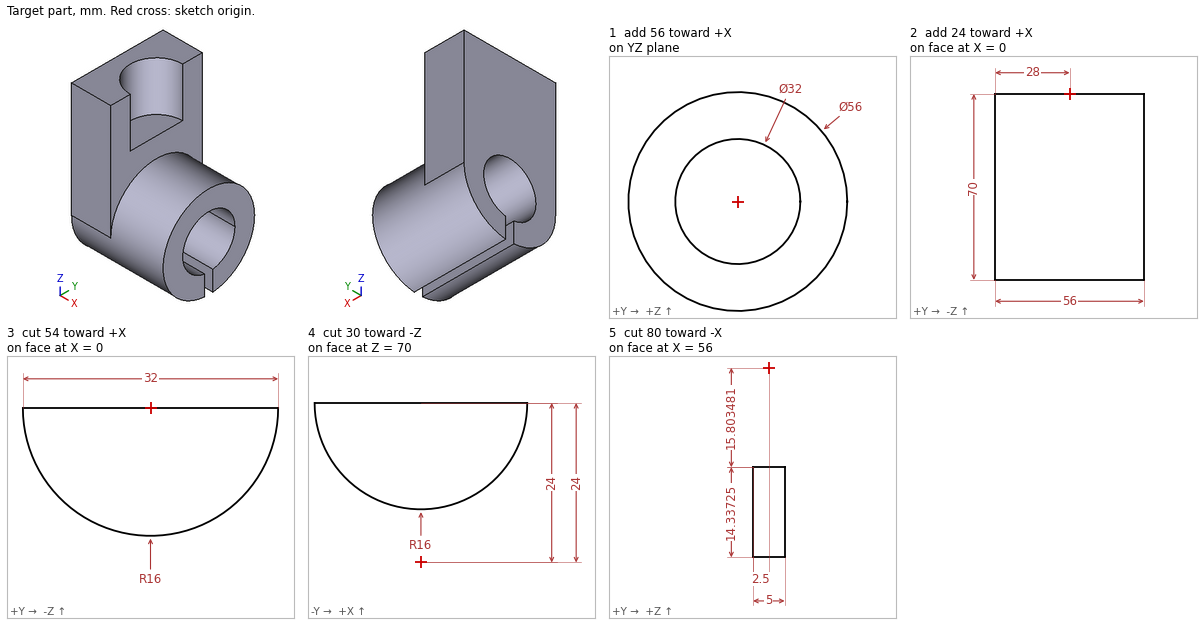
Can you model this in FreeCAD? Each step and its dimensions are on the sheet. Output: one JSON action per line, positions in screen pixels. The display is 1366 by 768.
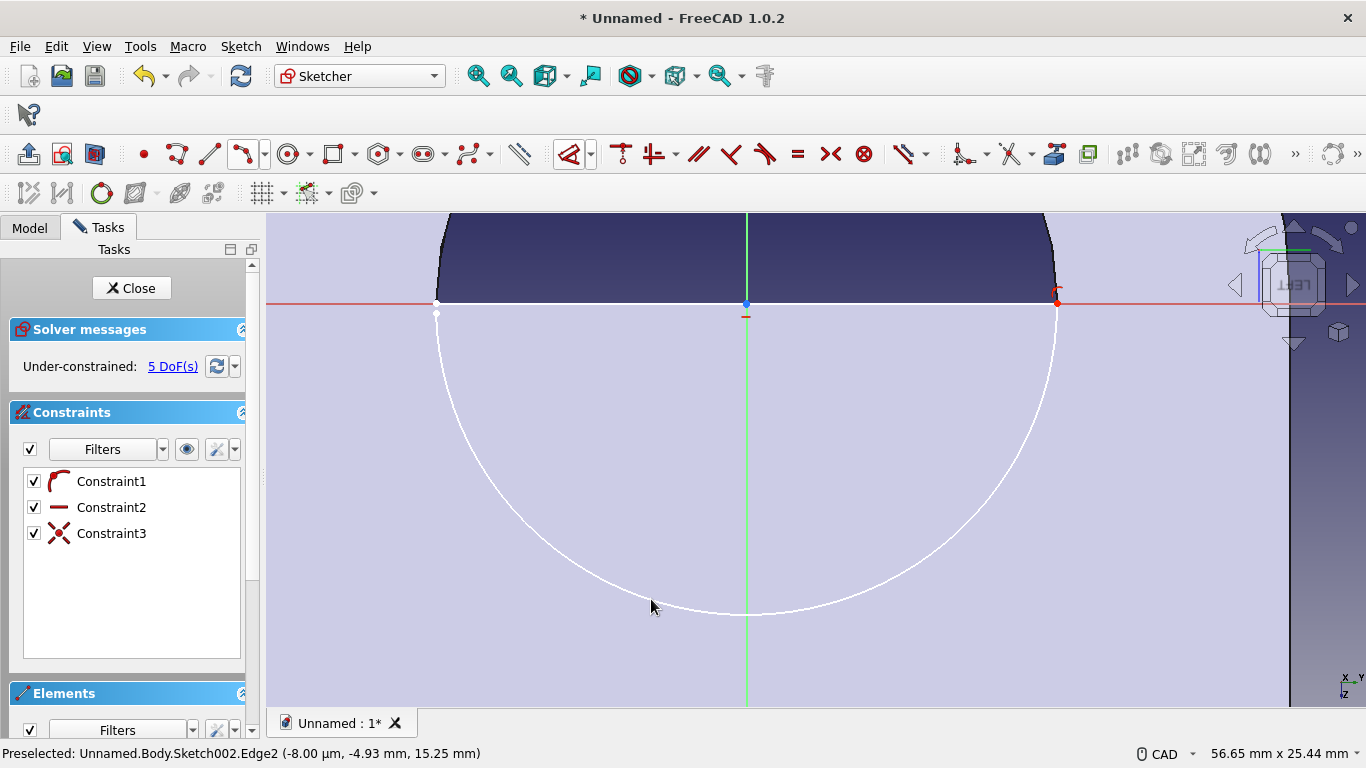
{"action": "left_click_drag", "start_coordinate": [736, 294], "coordinate": [757, 314]}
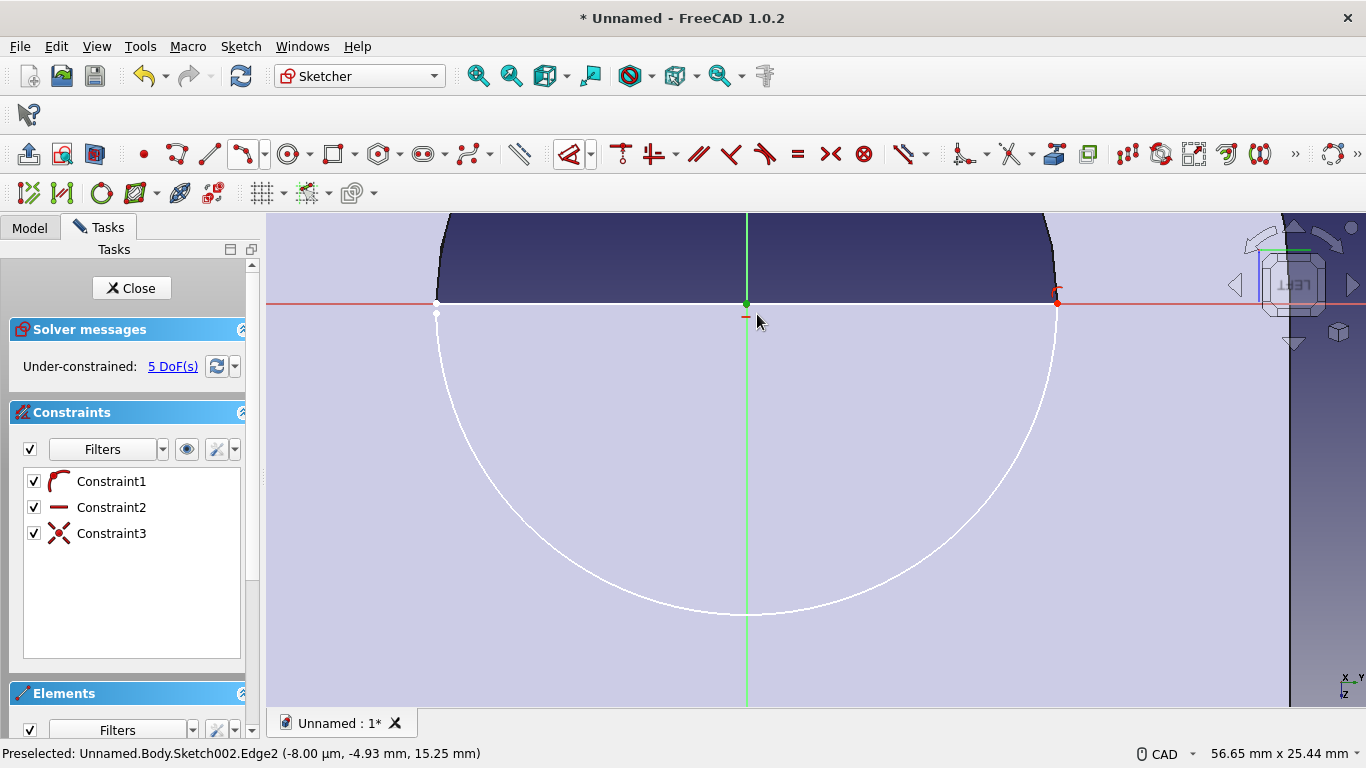
{"action": "left_click", "coordinate": [621, 154]}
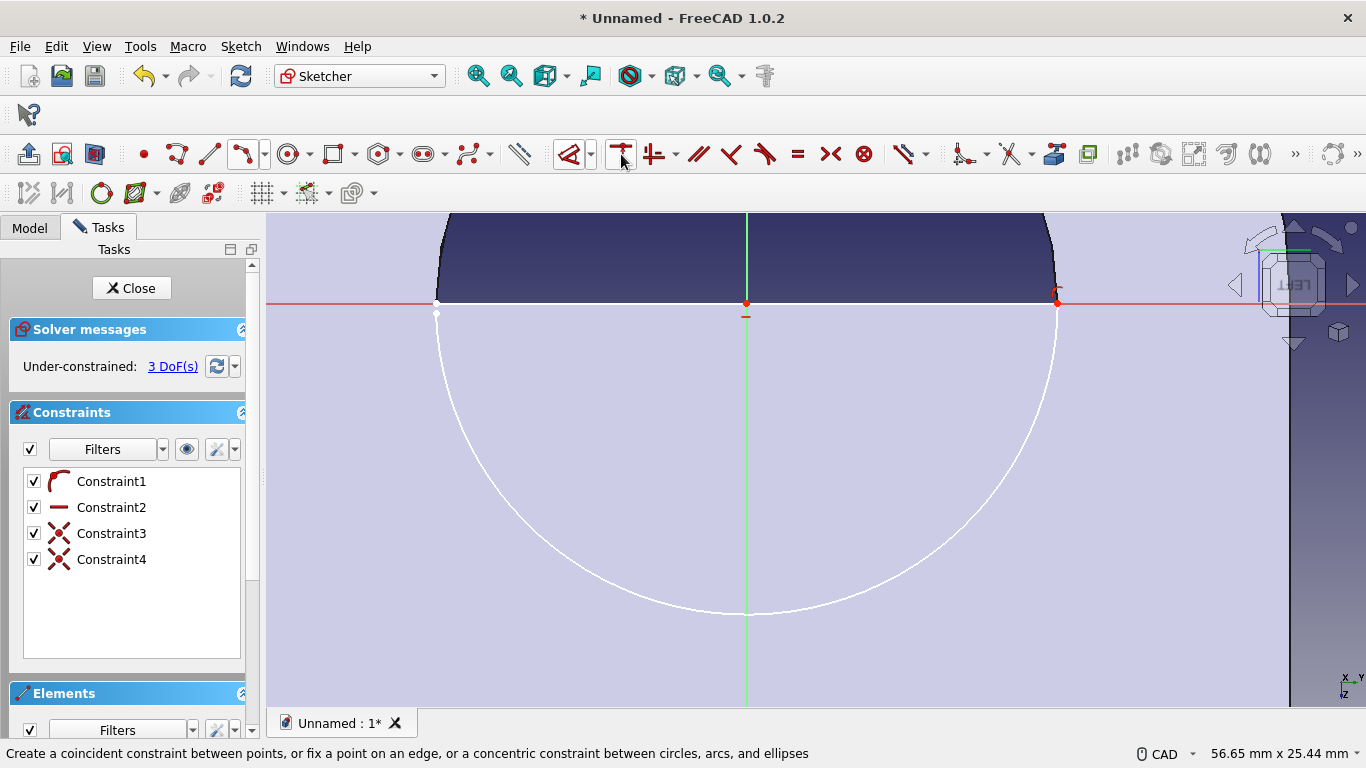
{"action": "left_click", "coordinate": [570, 559]}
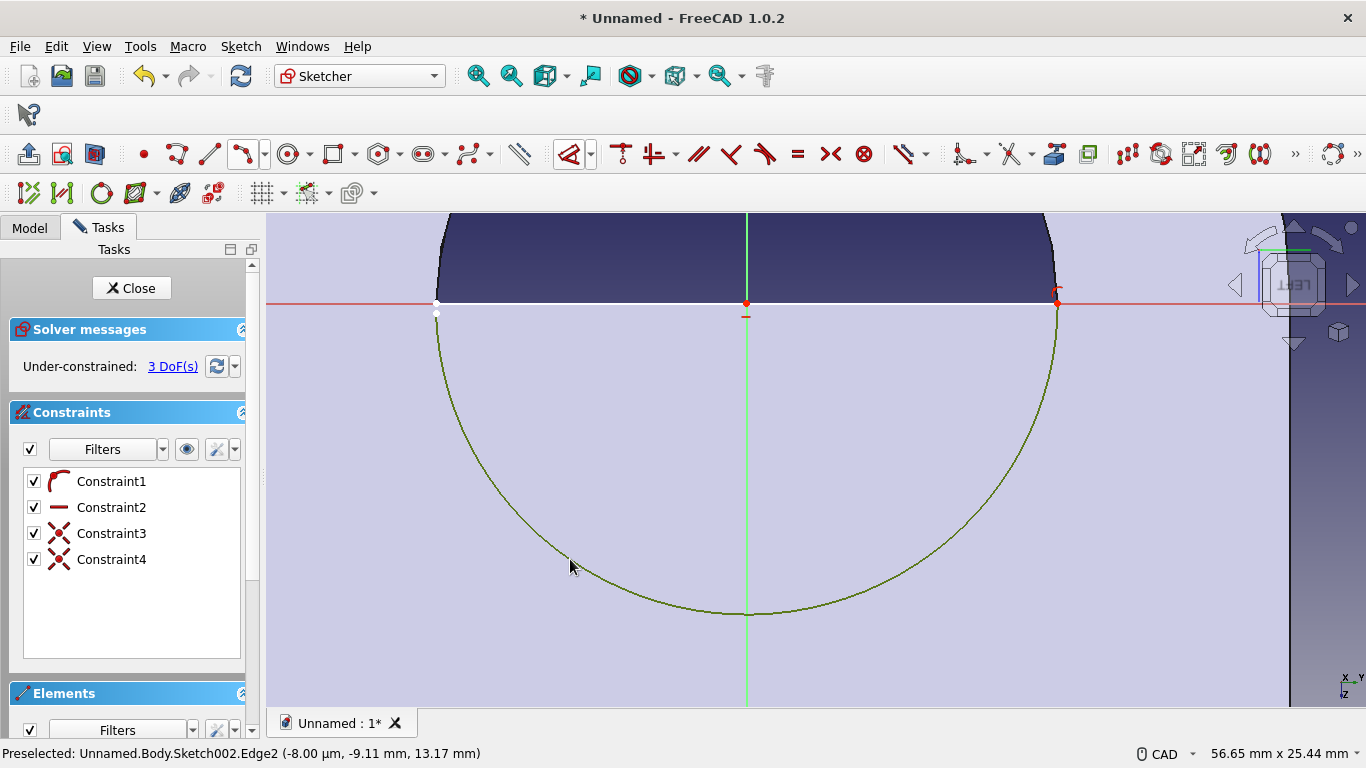
{"action": "key", "text": "k r"}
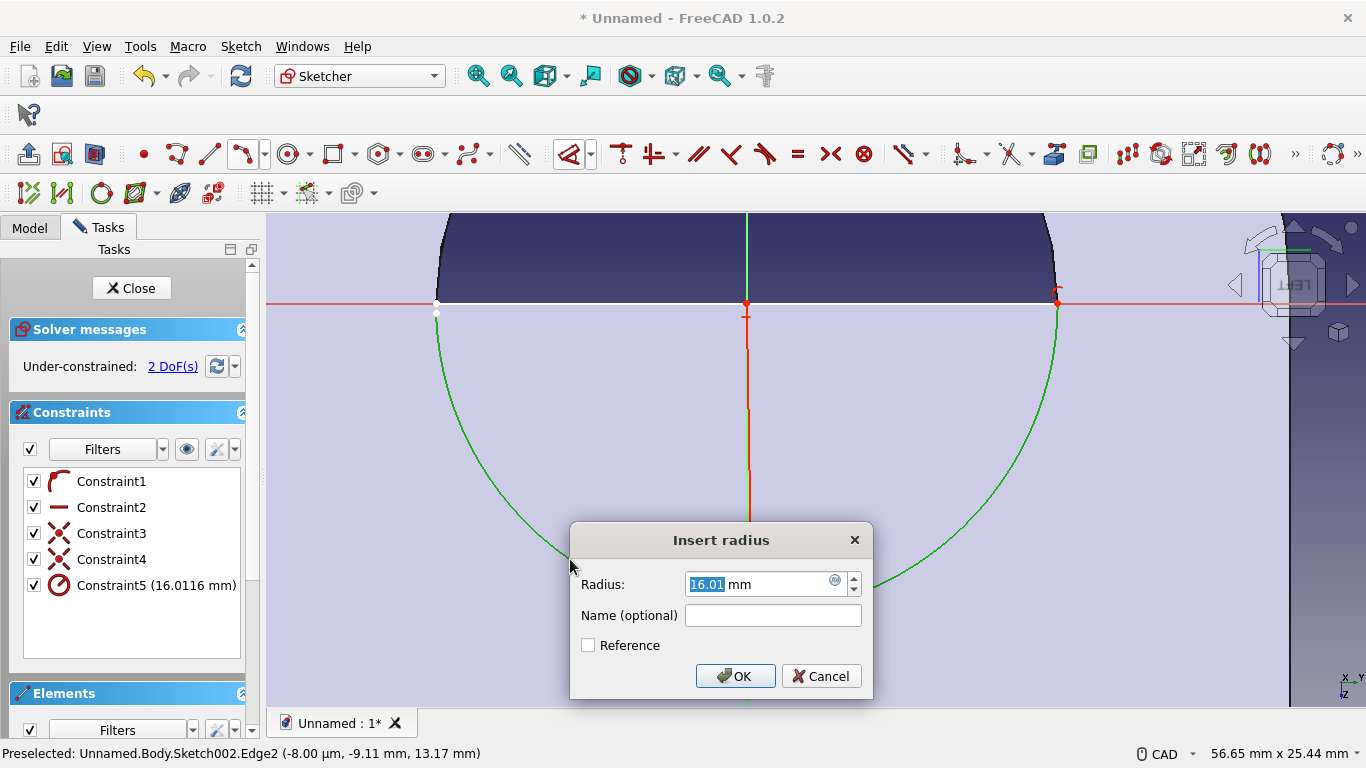
{"action": "type", "text": "16"}
{"action": "key", "text": "Return"}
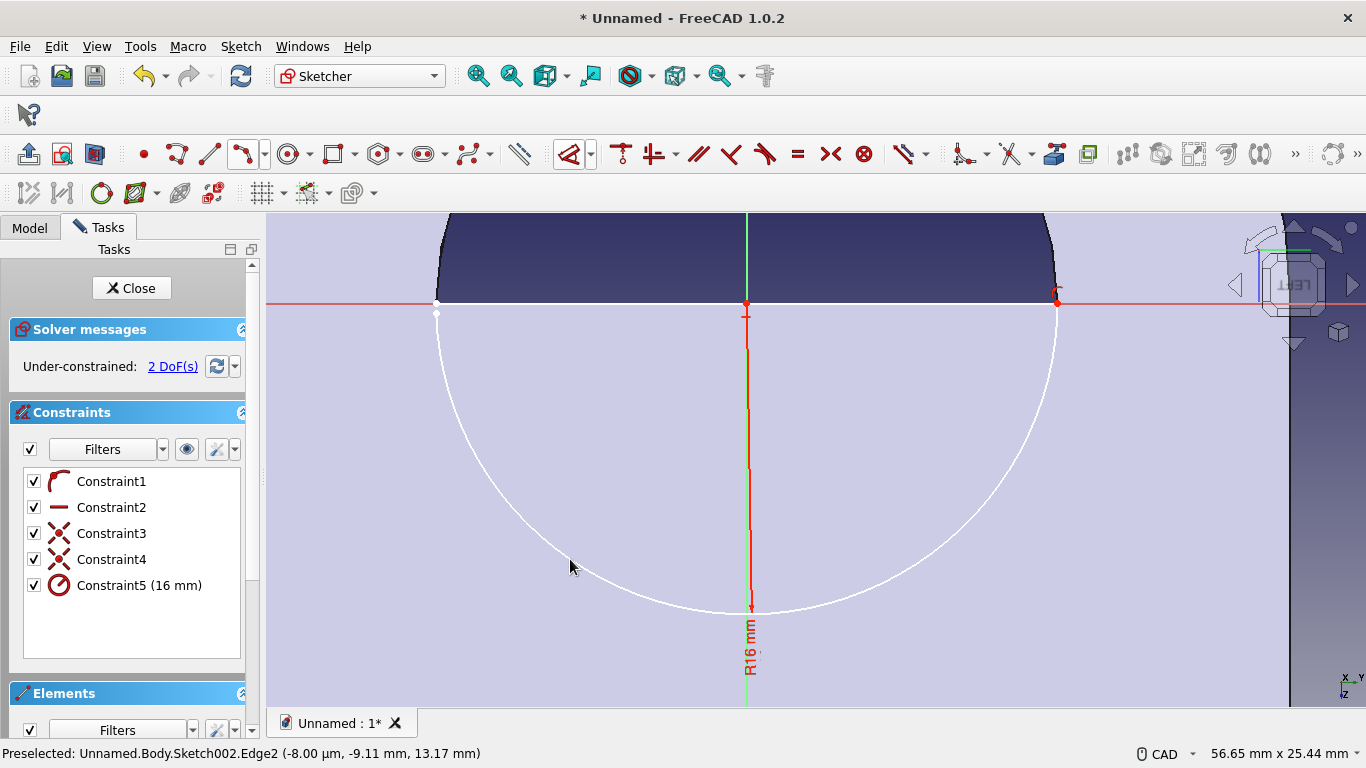
{"action": "left_click", "coordinate": [436, 314]}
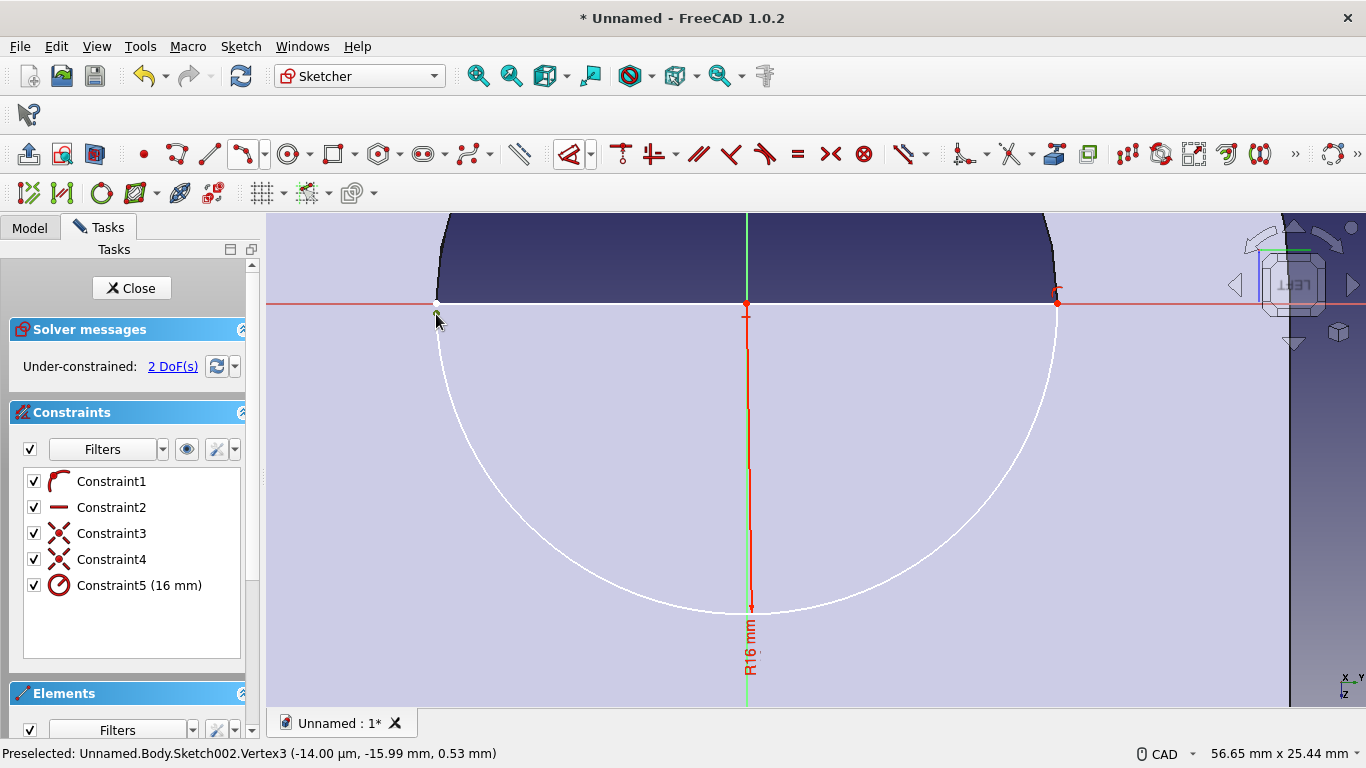
{"action": "left_click", "coordinate": [359, 304]}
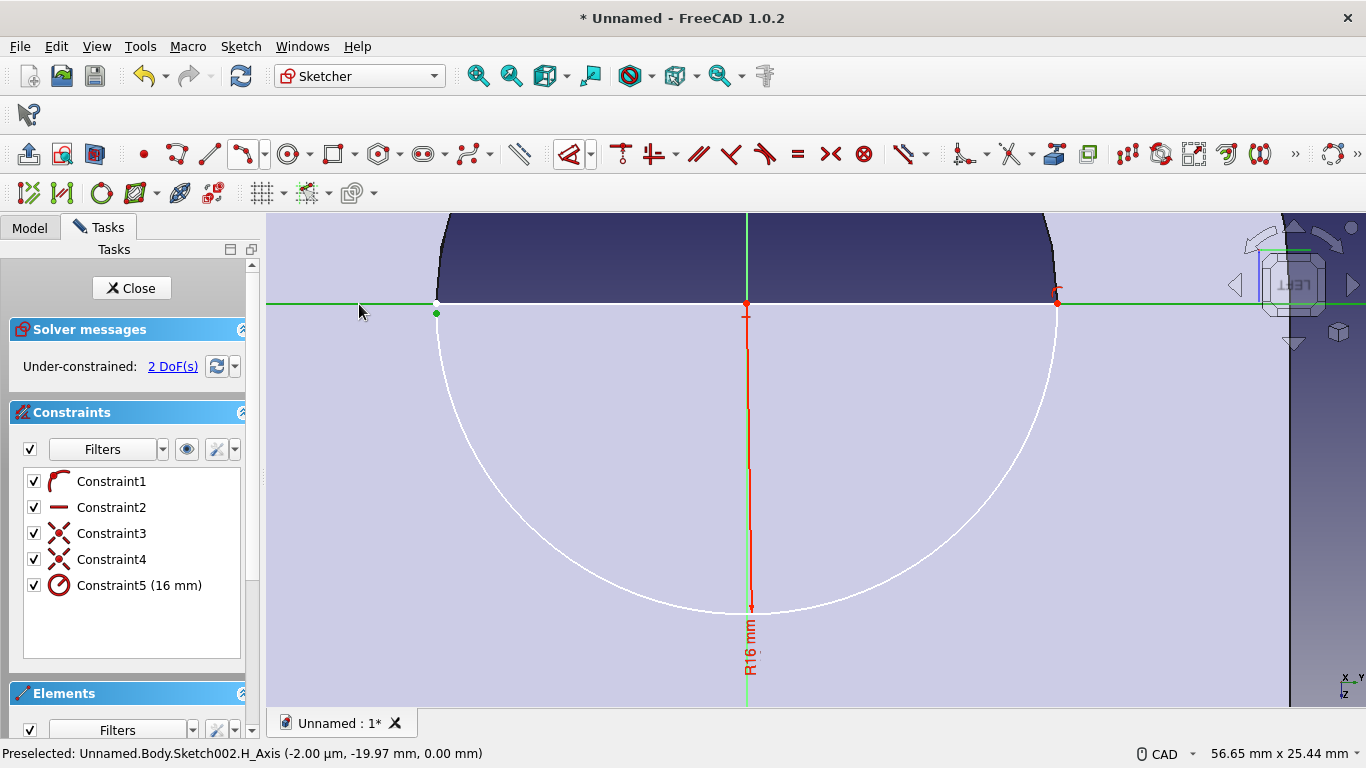
{"action": "left_click", "coordinate": [621, 154]}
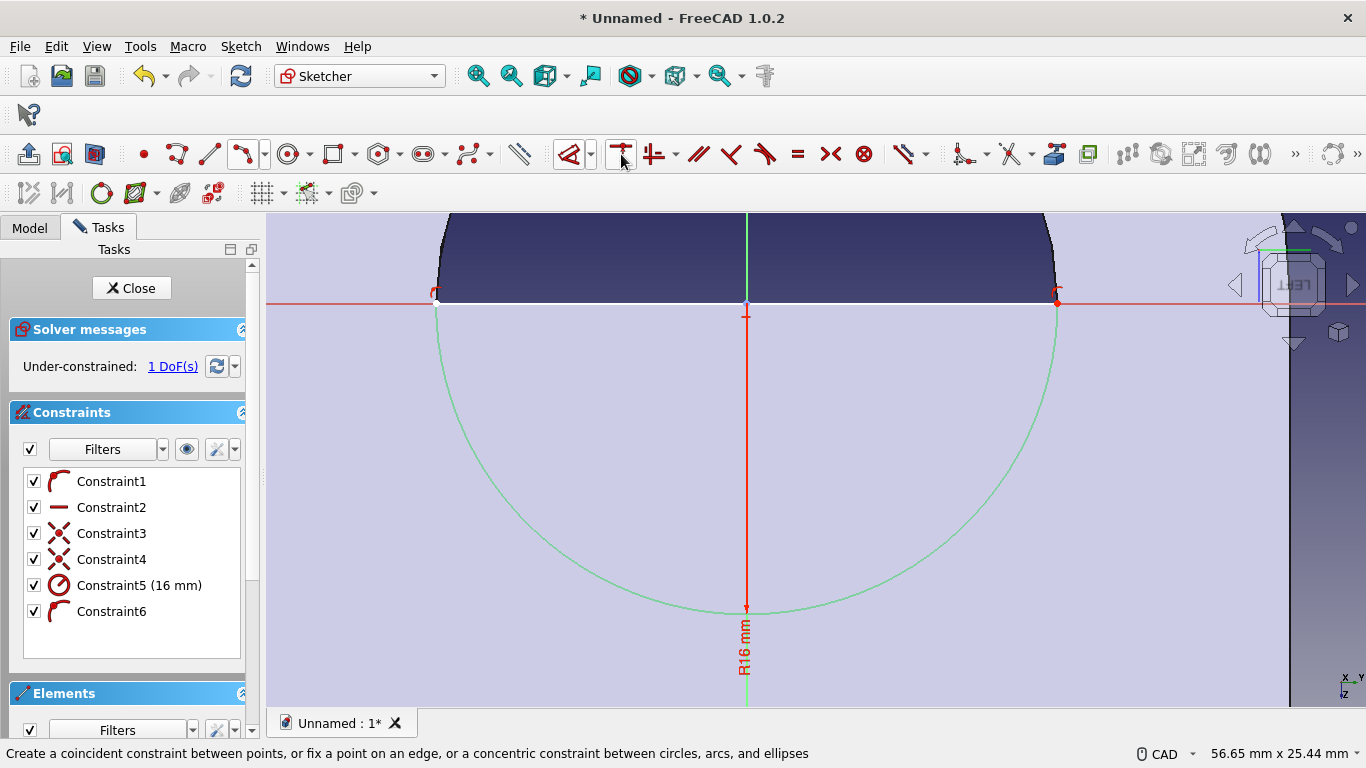
{"action": "left_click", "coordinate": [871, 304]}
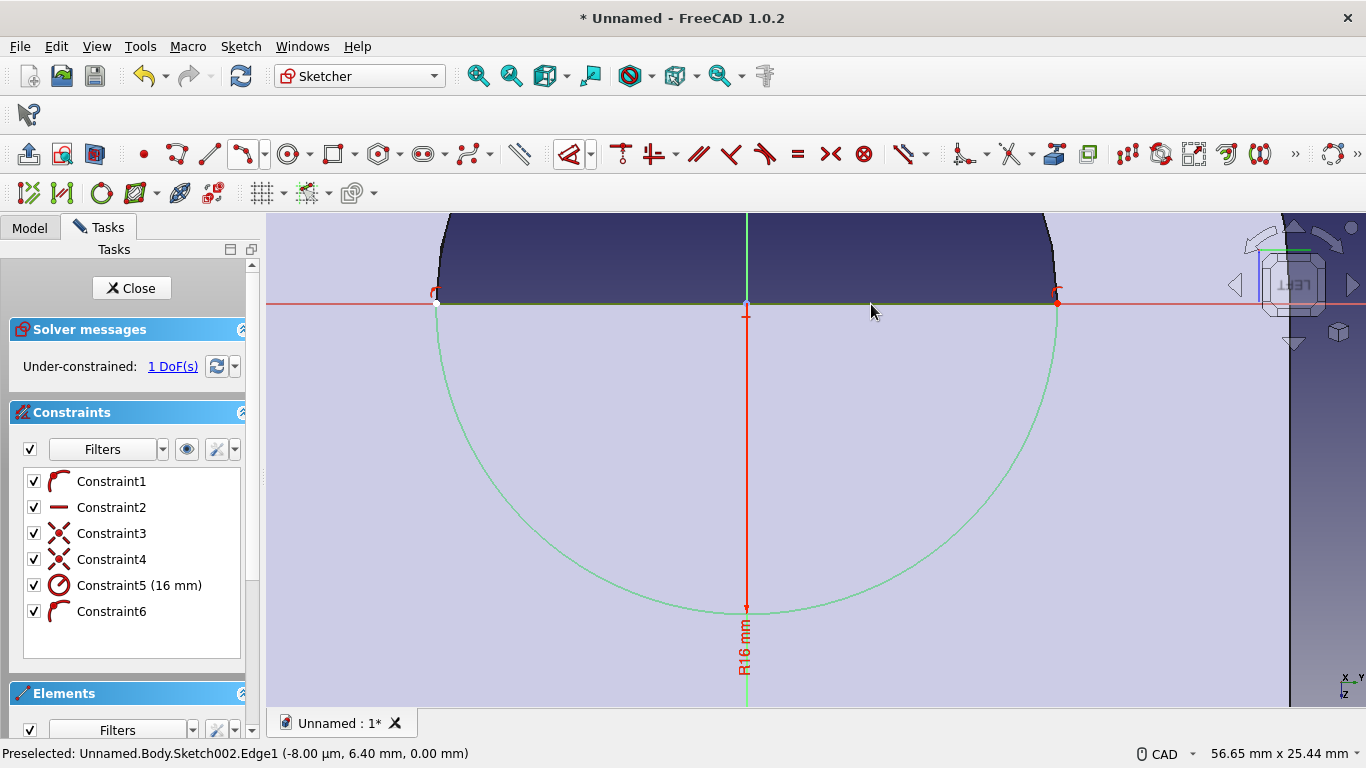
{"action": "key", "text": "l"}